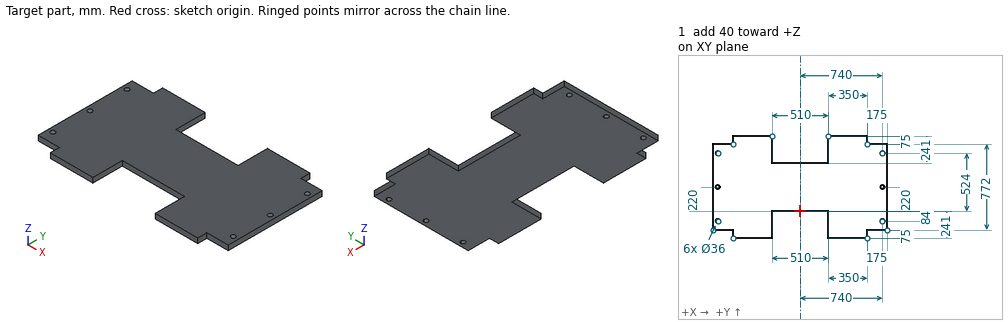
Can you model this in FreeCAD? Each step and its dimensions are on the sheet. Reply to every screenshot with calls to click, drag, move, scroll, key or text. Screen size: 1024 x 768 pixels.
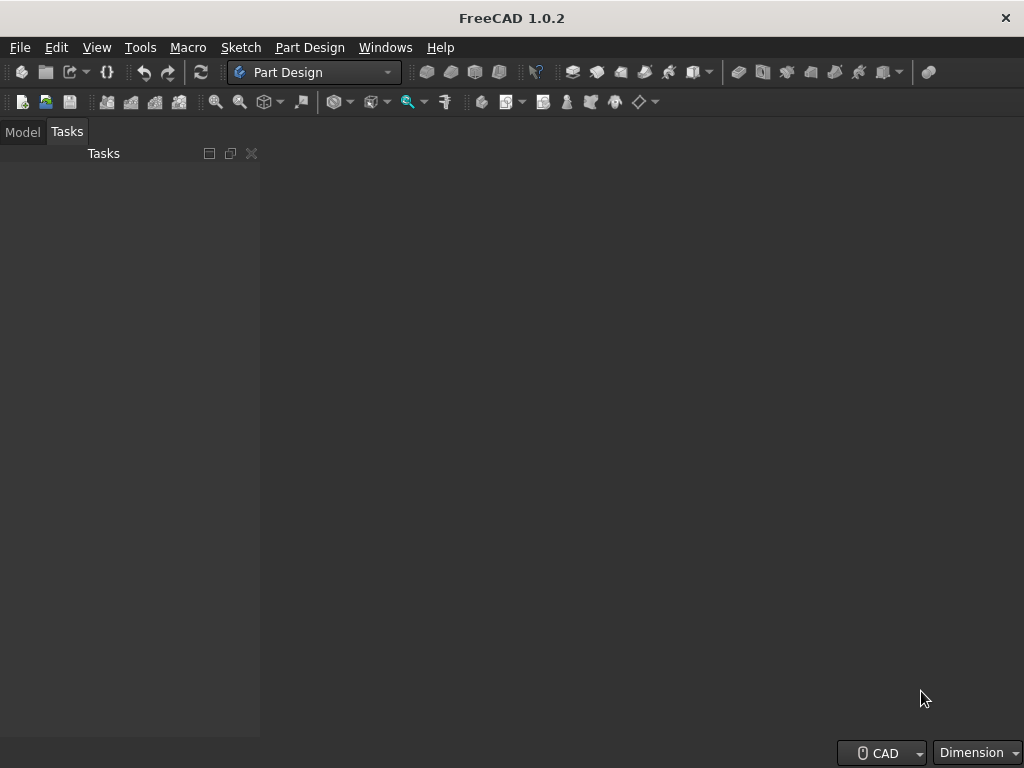
click(22, 102)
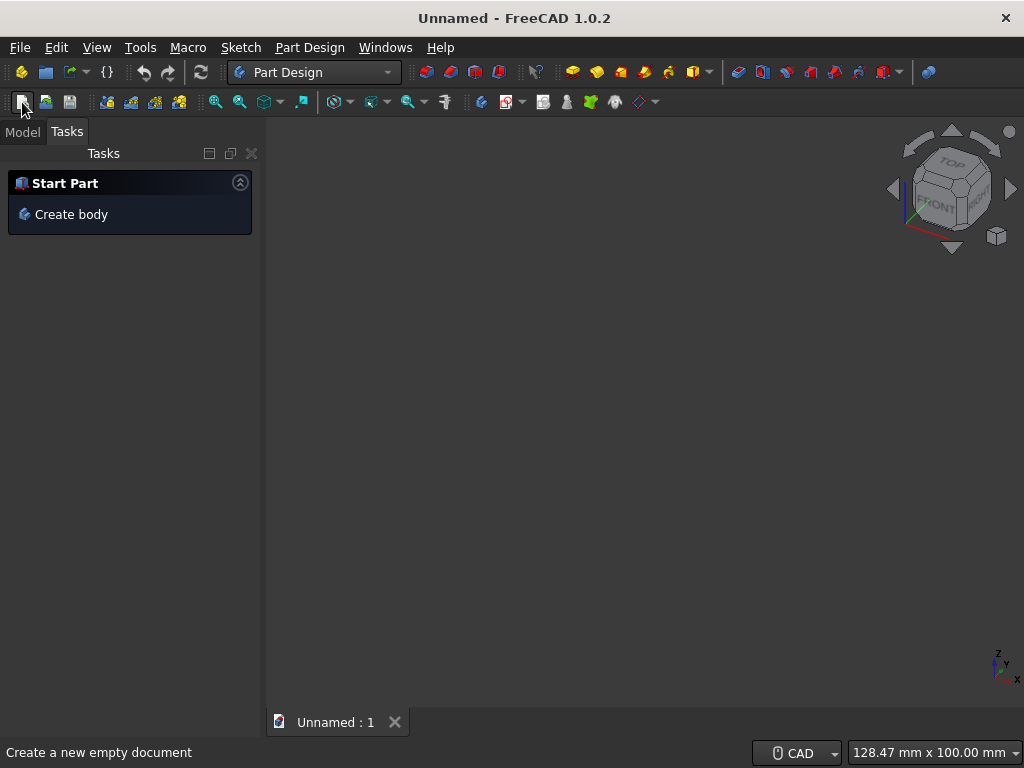
click(506, 102)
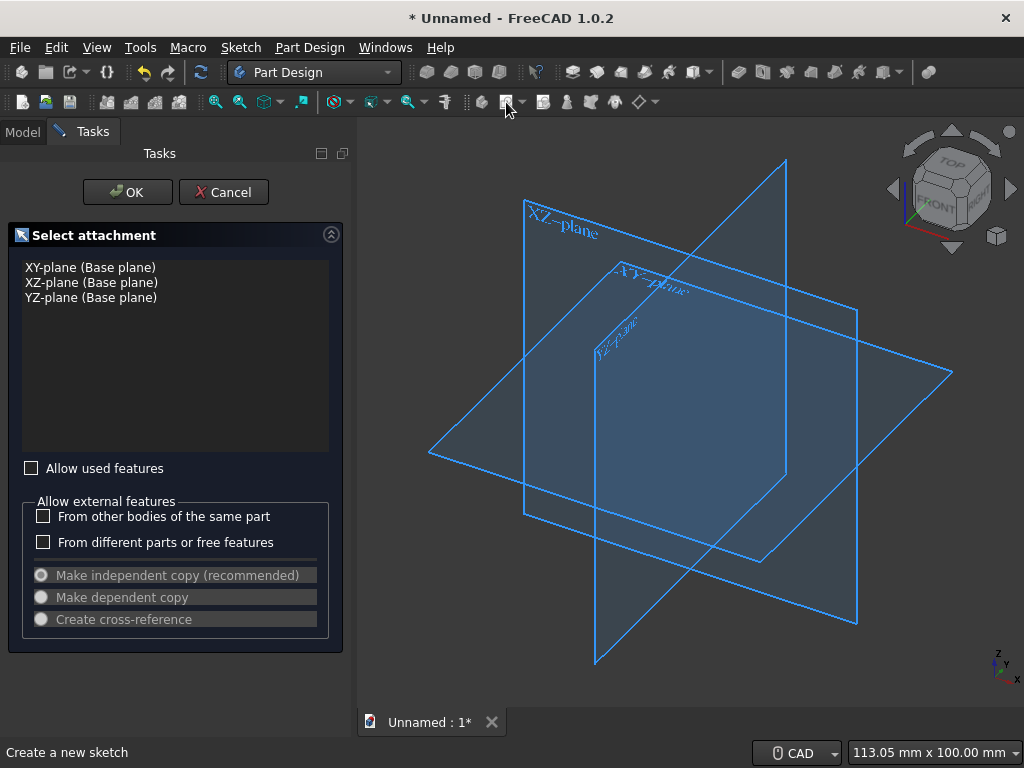
click(82, 268)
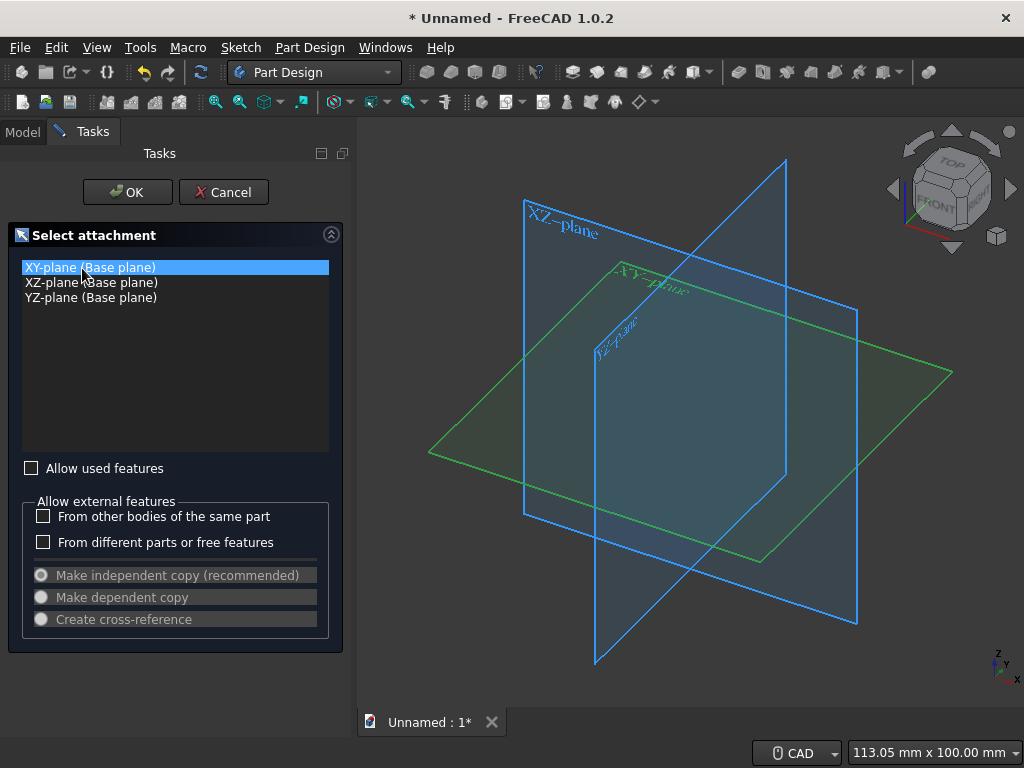
click(128, 192)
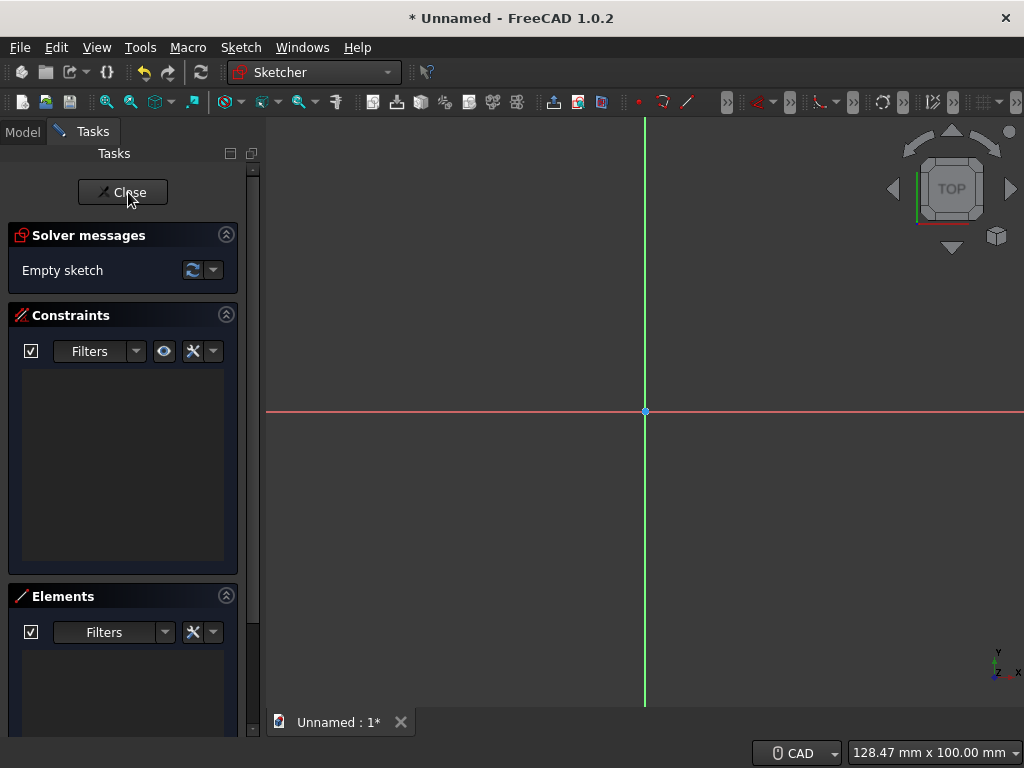
scroll(573, 480, down, 15)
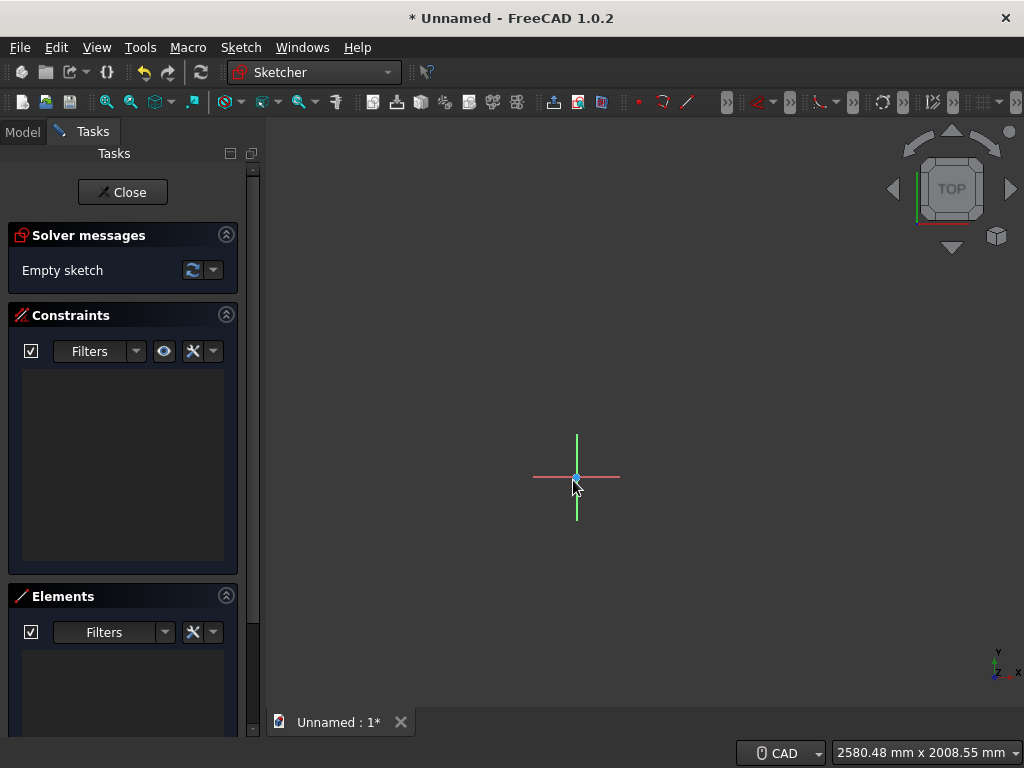
click(664, 102)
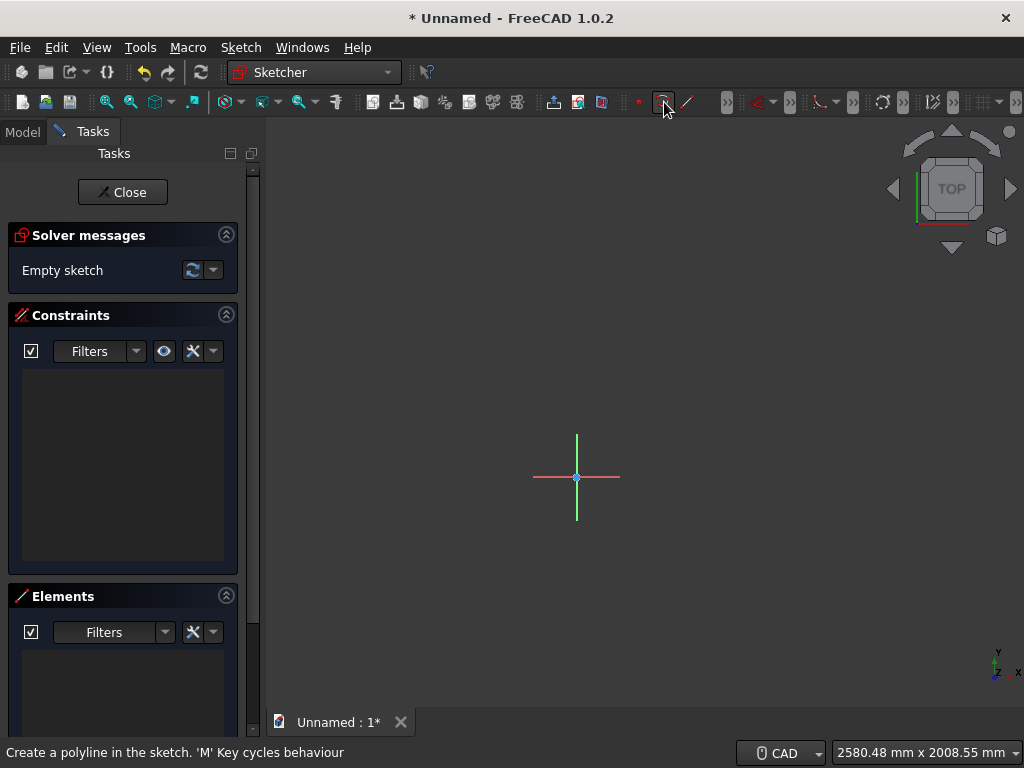
click(502, 477)
click(652, 468)
click(652, 548)
click(755, 548)
click(755, 526)
click(806, 526)
click(806, 299)
click(755, 299)
click(755, 277)
click(652, 277)
click(652, 348)
click(502, 348)
click(502, 277)
click(399, 277)
click(399, 299)
click(348, 299)
click(348, 526)
click(399, 526)
click(399, 548)
click(502, 548)
click(502, 478)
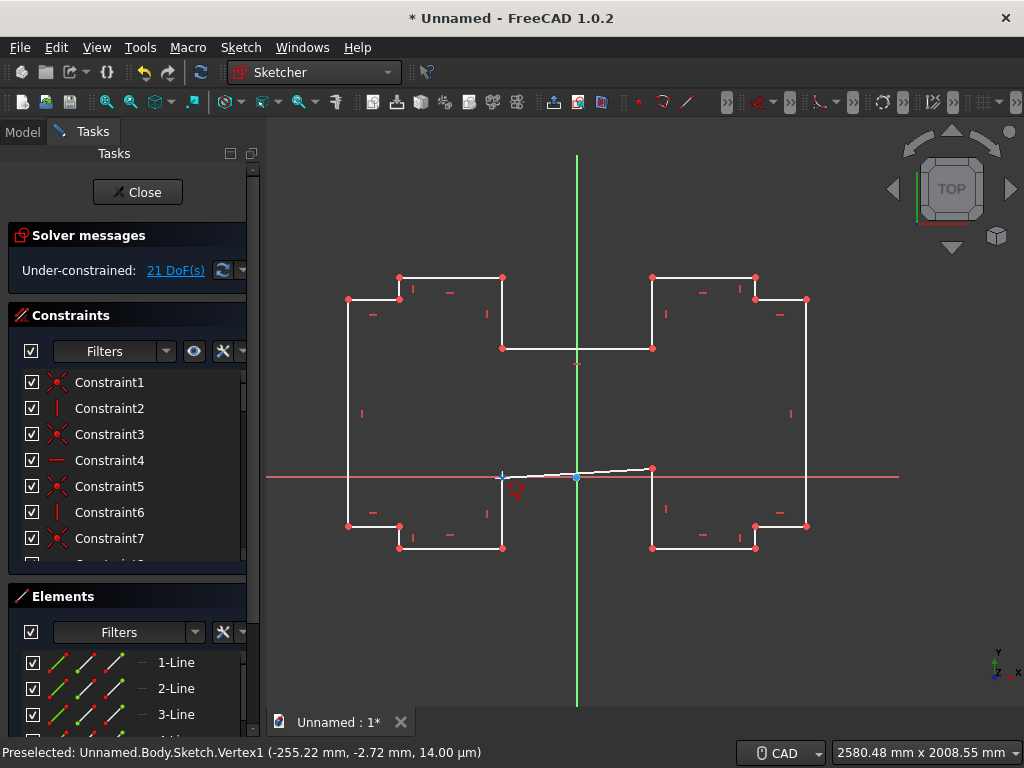
key(g)
key(c)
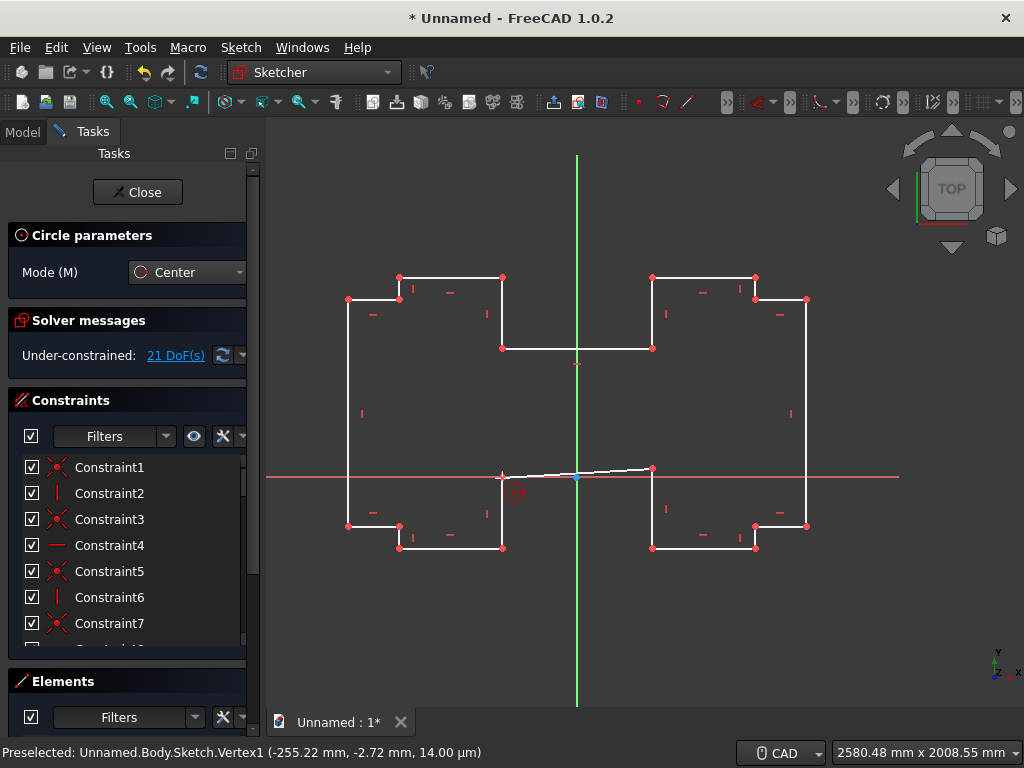
scroll(794, 502, up, 8)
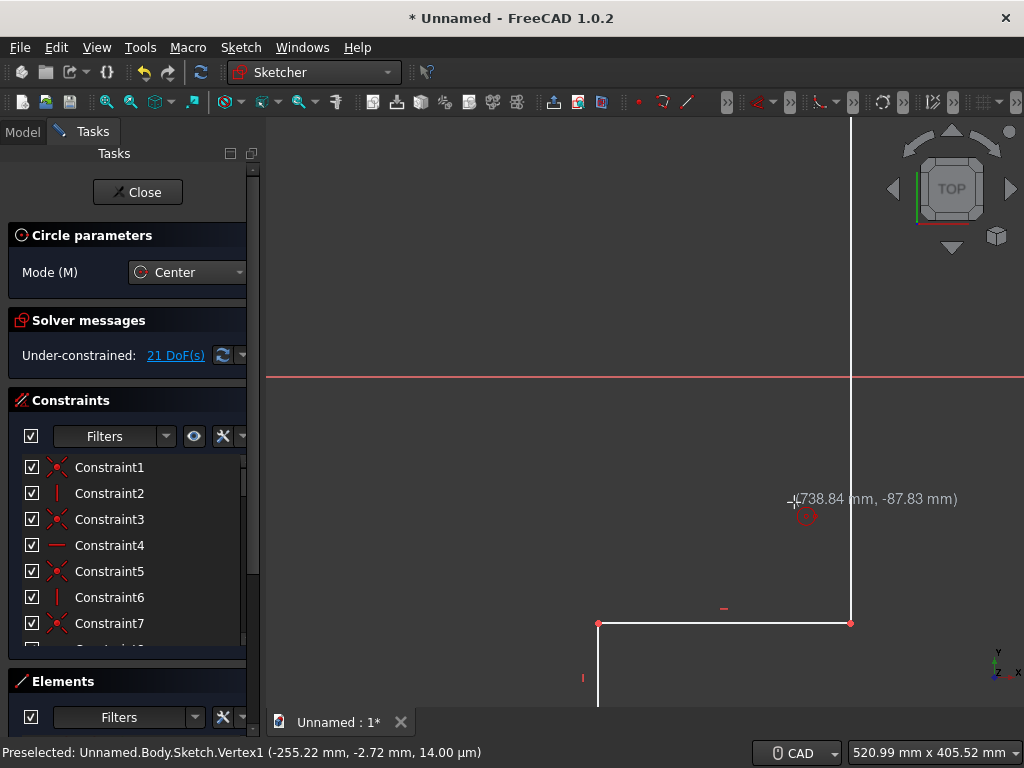
scroll(747, 482, down, 9)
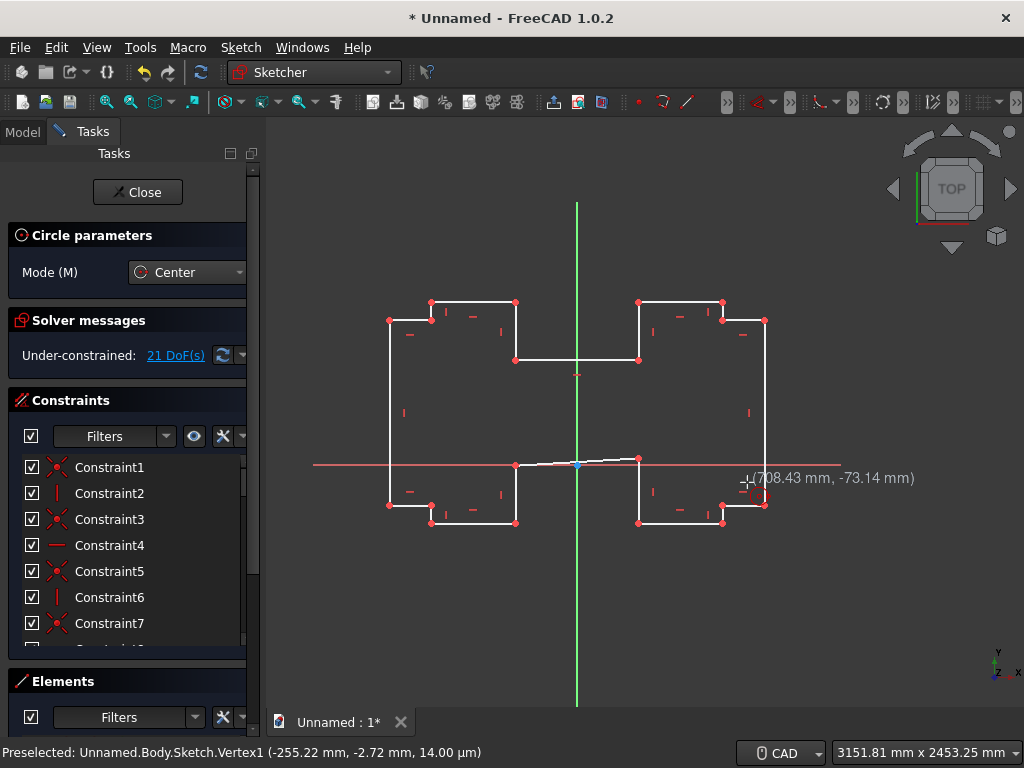
scroll(755, 485, up, 3)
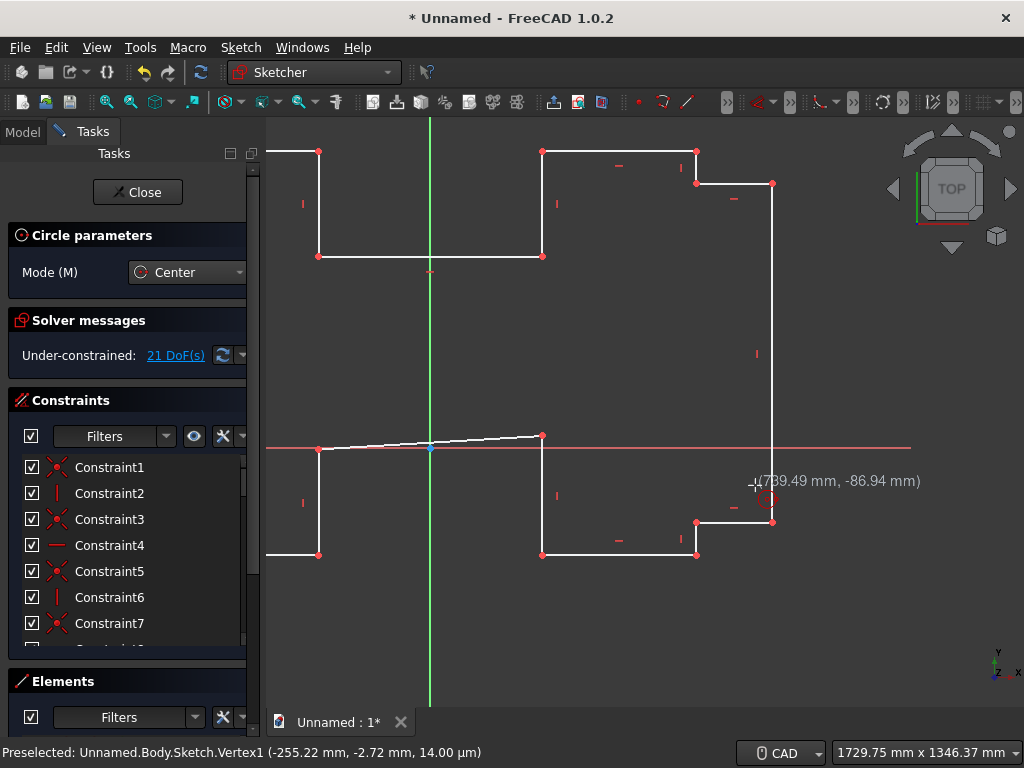
click(755, 485)
move(749, 479)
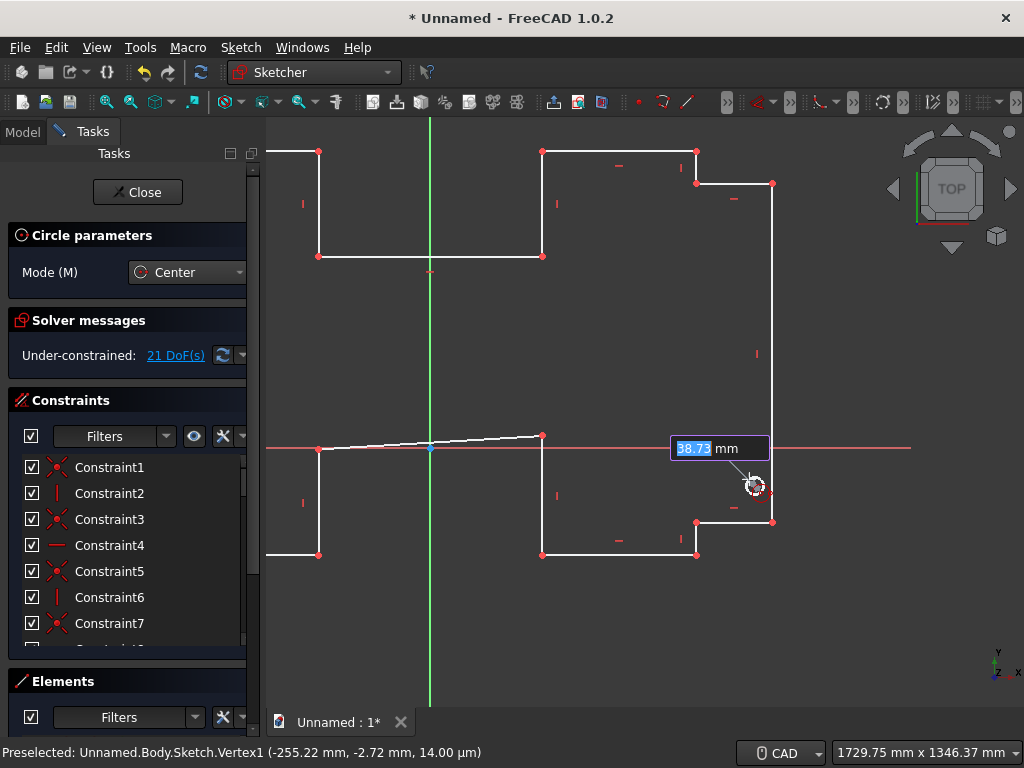
text(36)
key(Return)